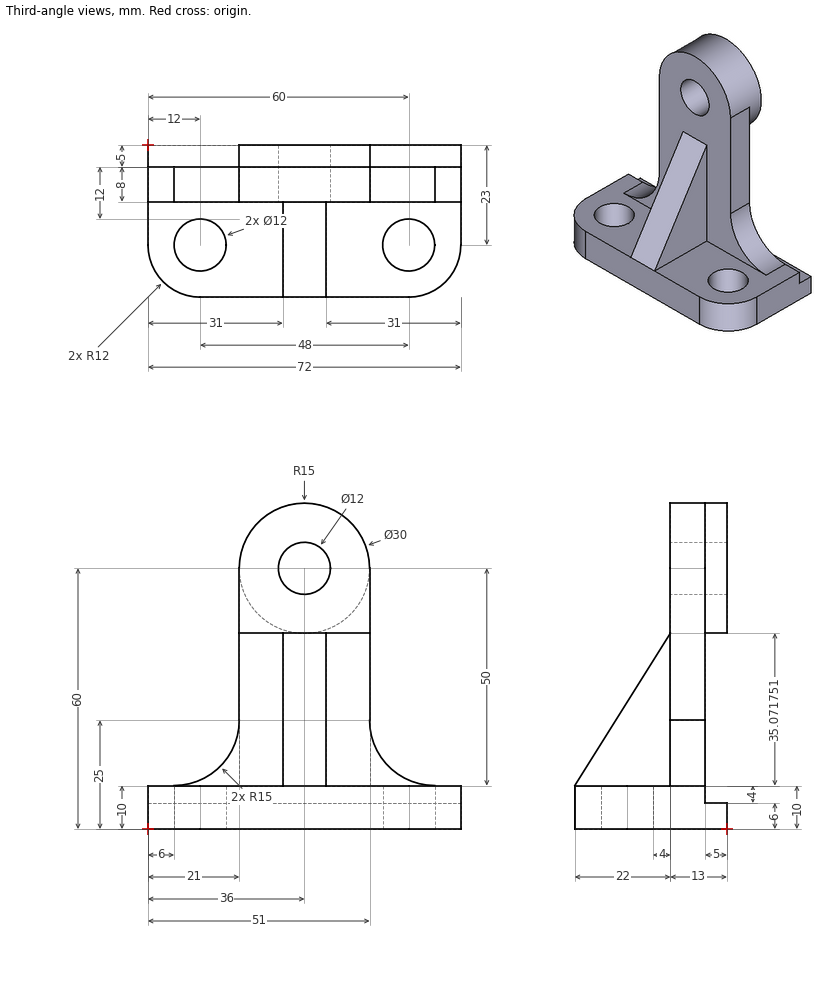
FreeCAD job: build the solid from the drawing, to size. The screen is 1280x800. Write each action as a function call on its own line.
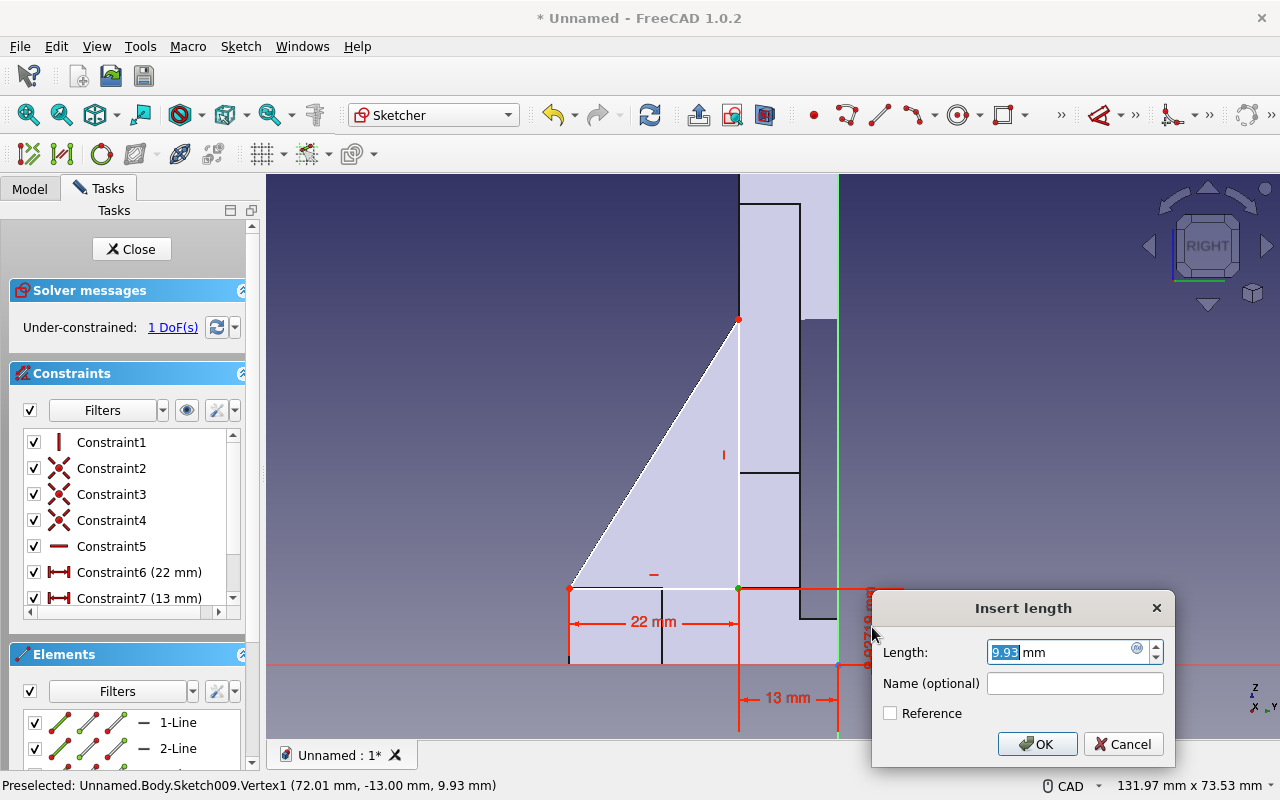
text(10)
key(Return)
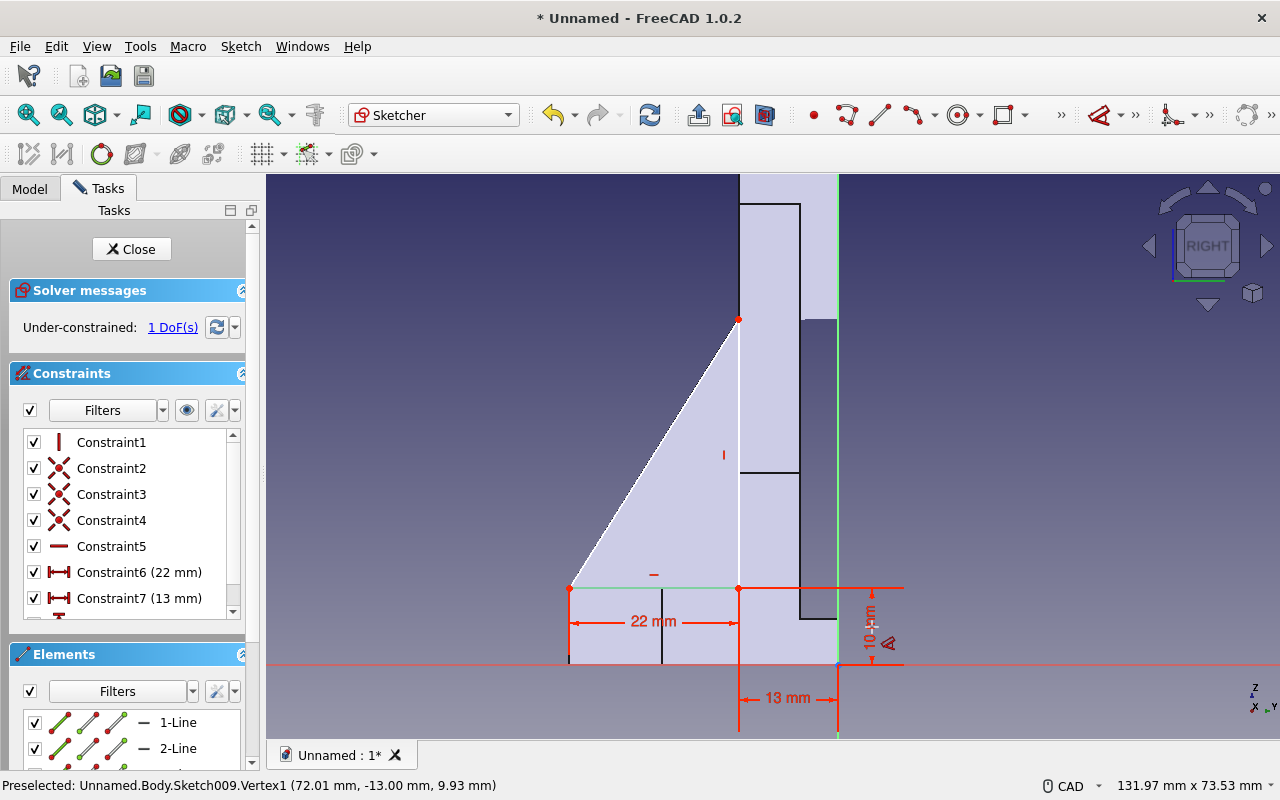
click(739, 508)
click(773, 454)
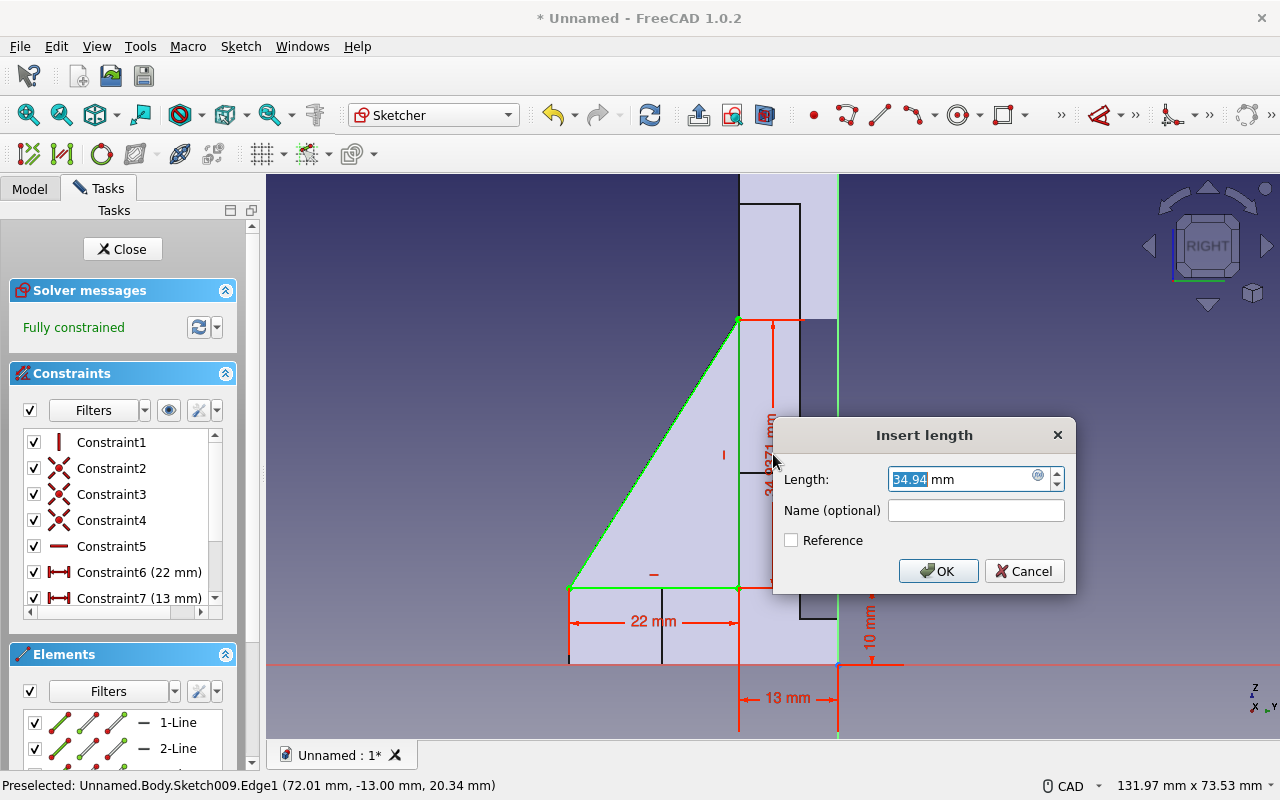
text(35.071751)
key(Return)
key(Escape)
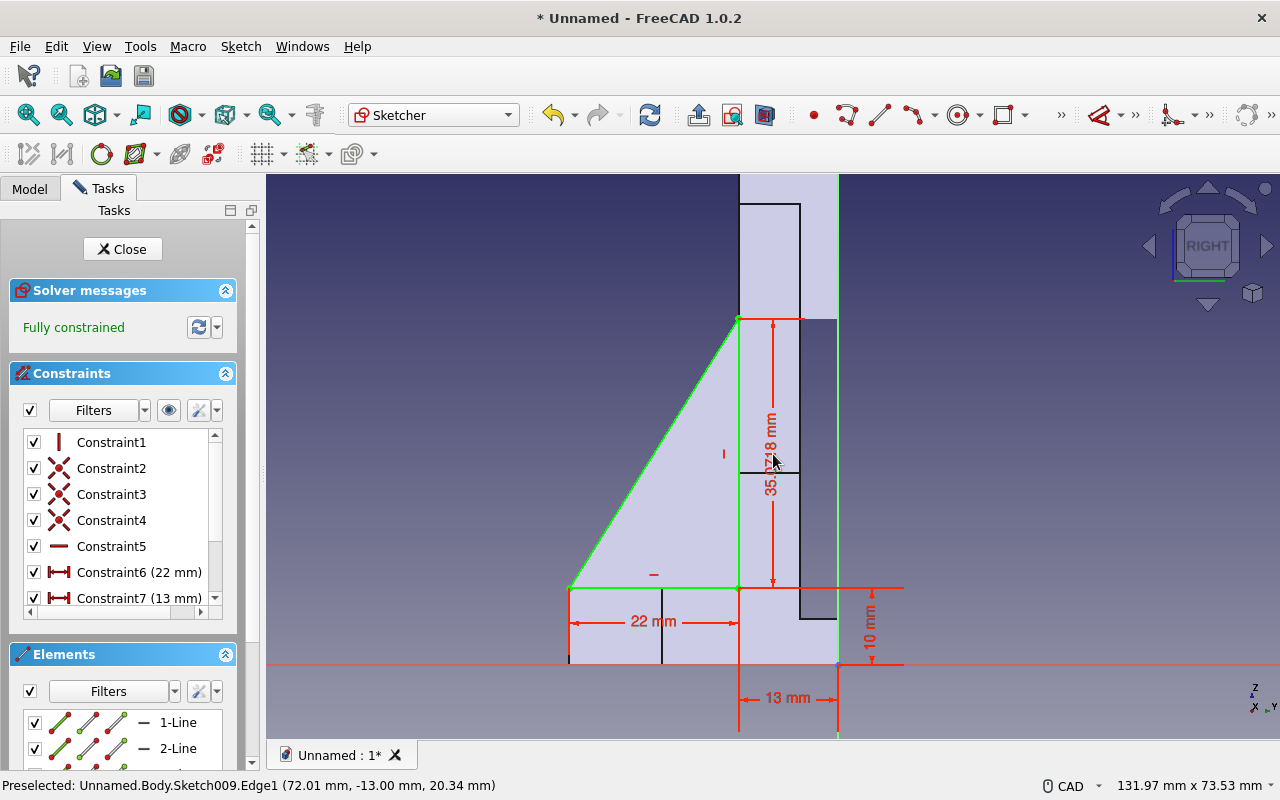
click(123, 249)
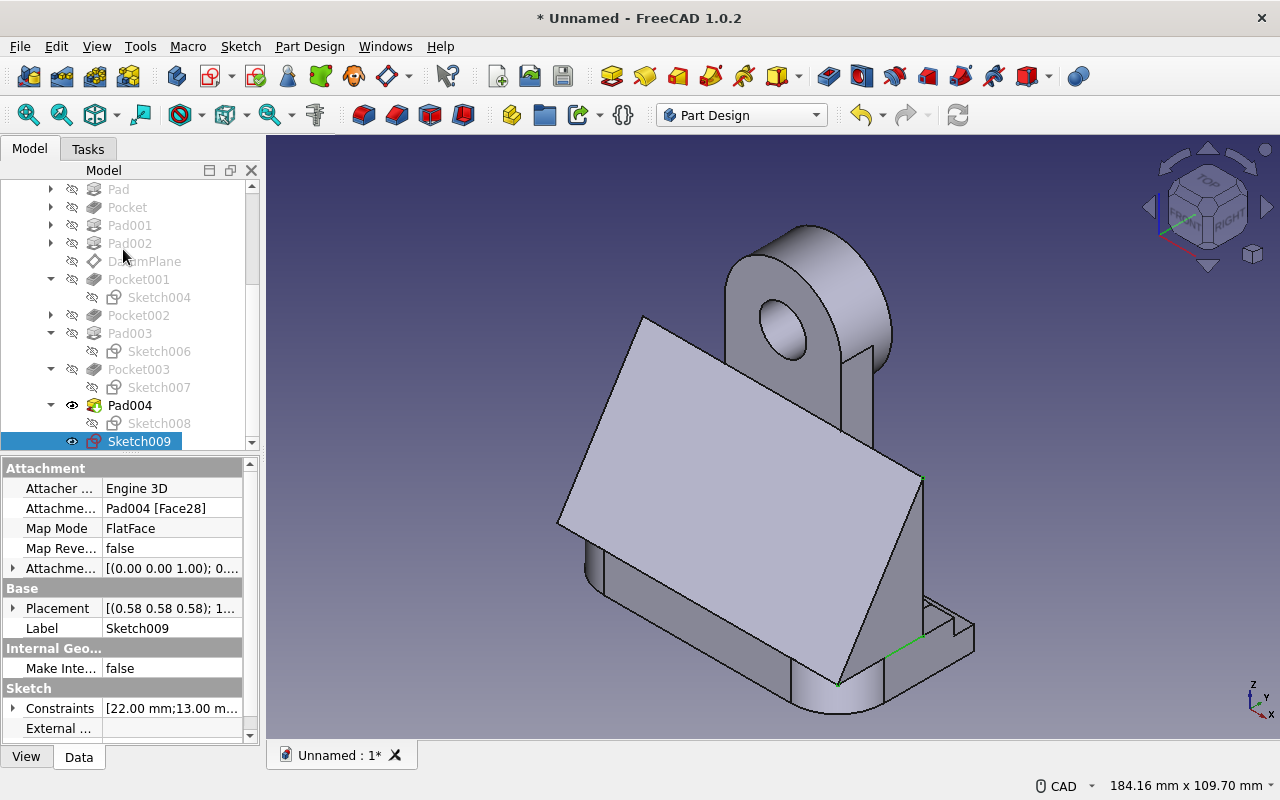
click(829, 76)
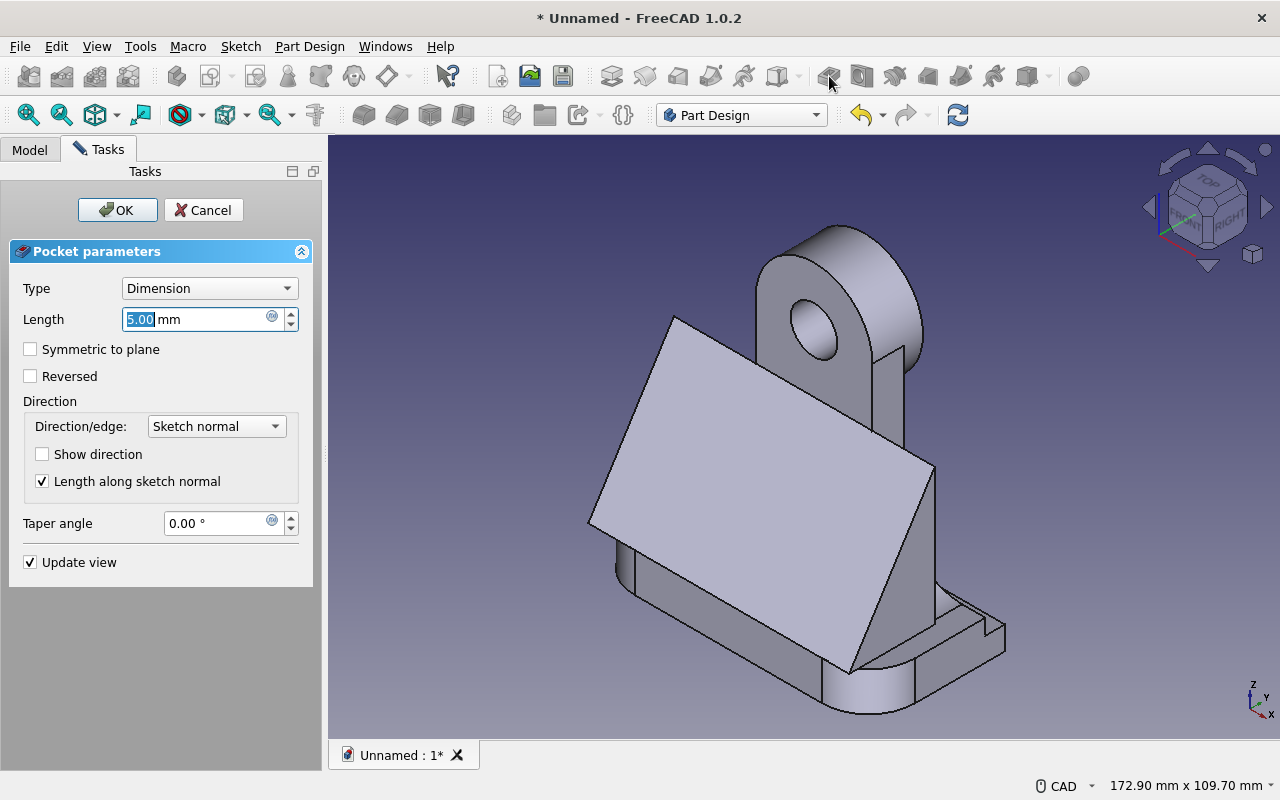
text(31)
key(Tab)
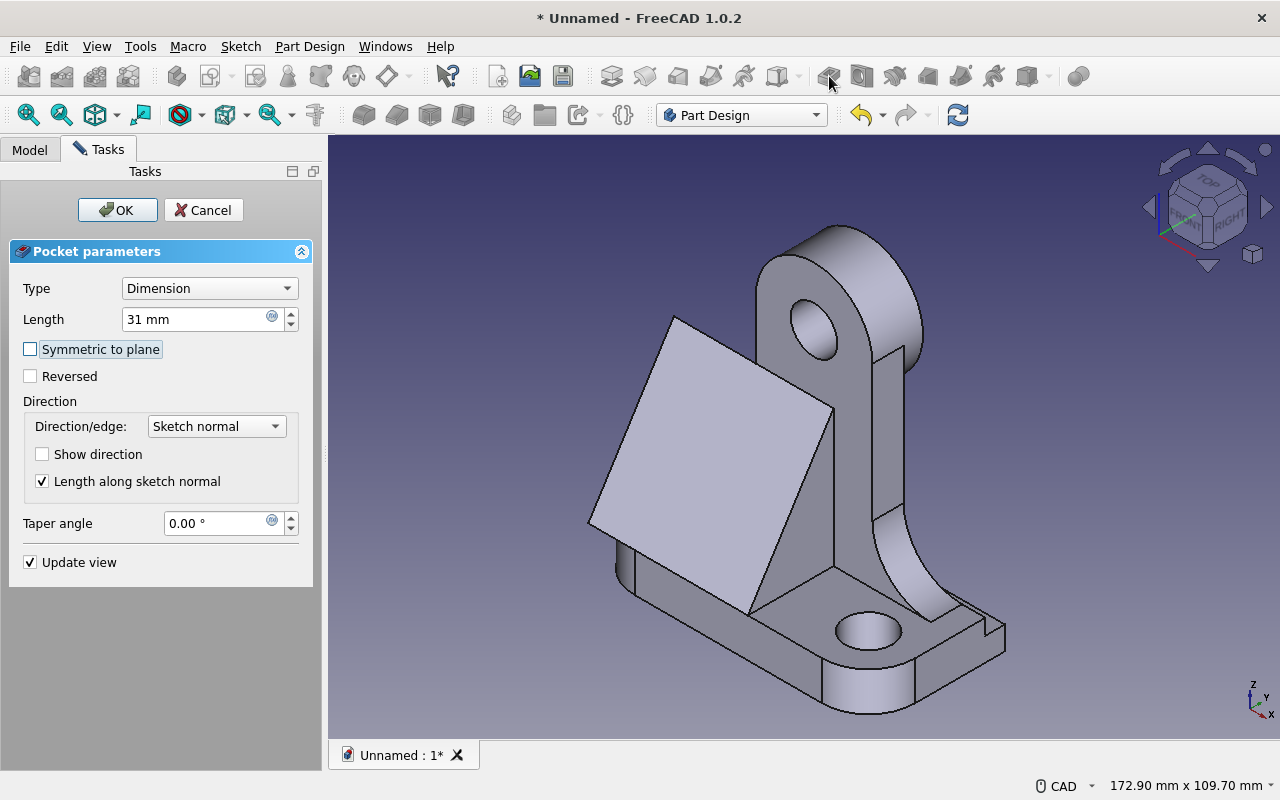
click(118, 210)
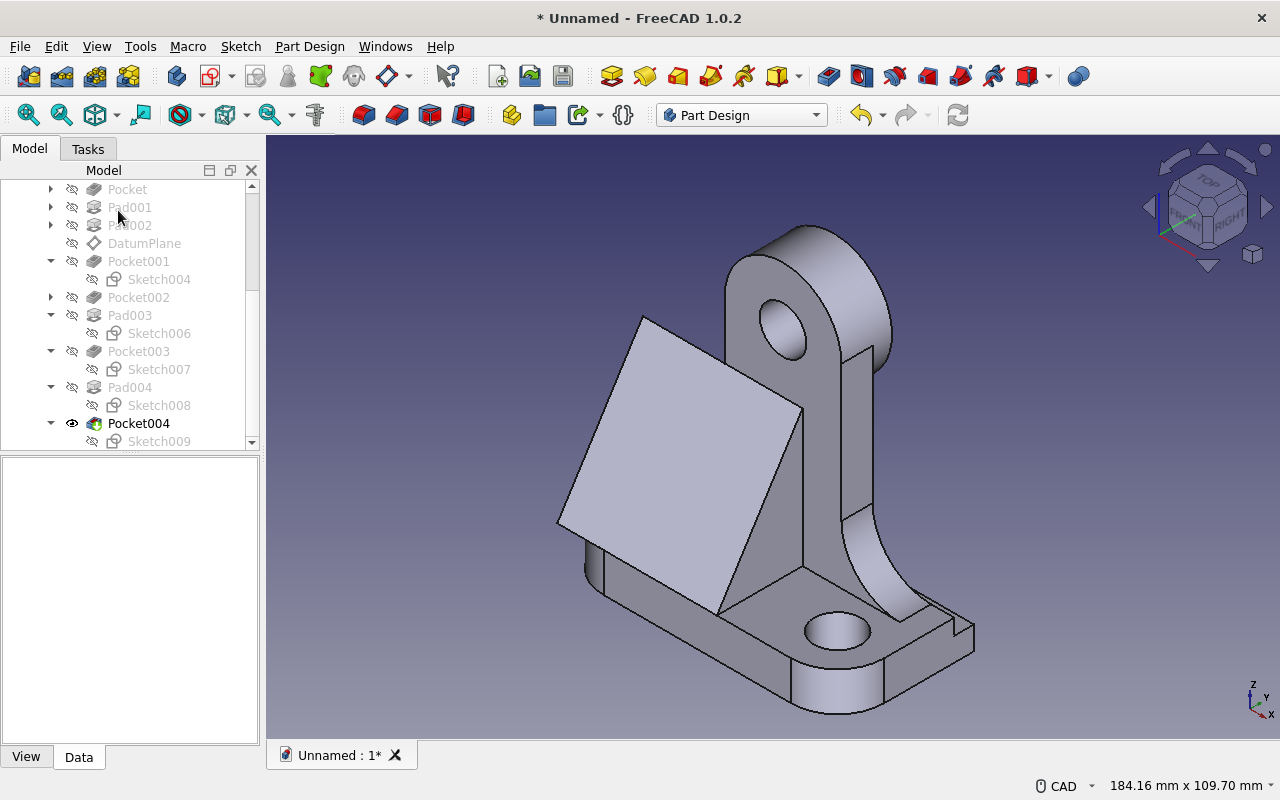
key(6)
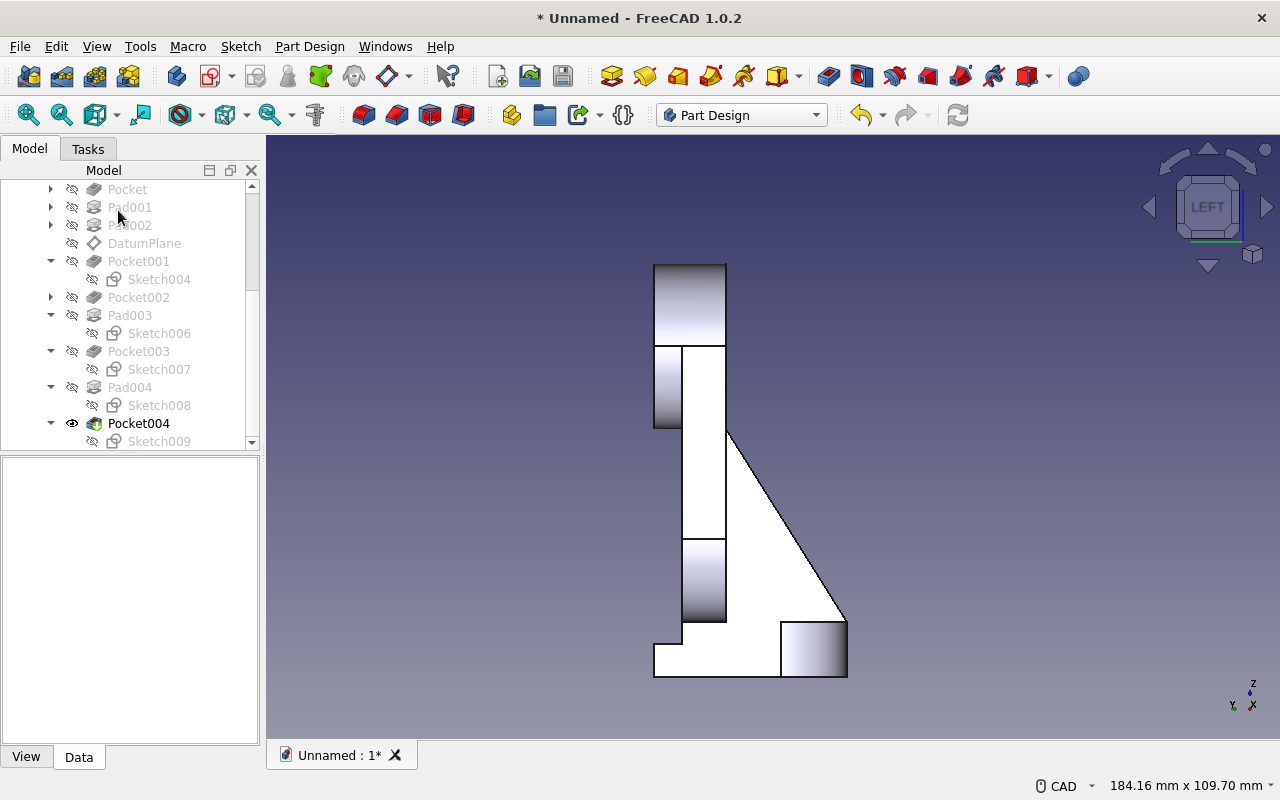
click(778, 587)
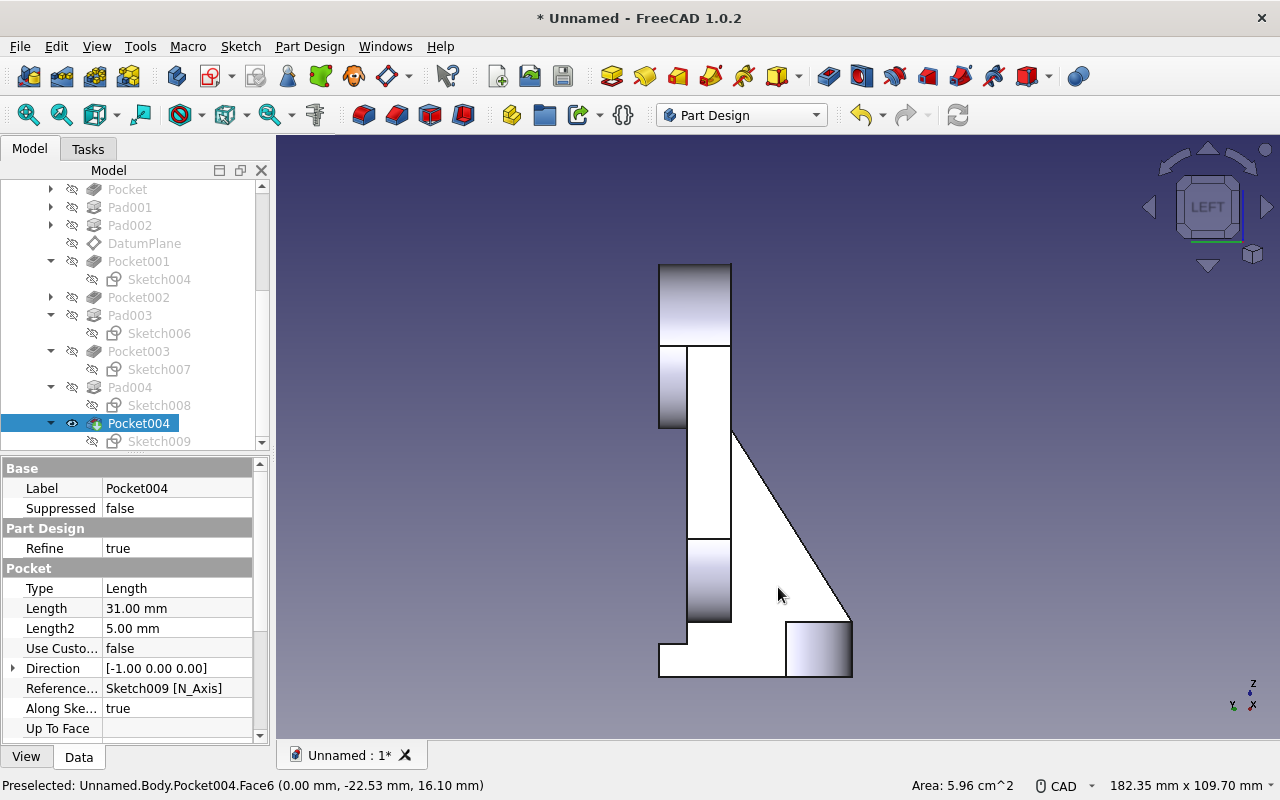
click(210, 76)